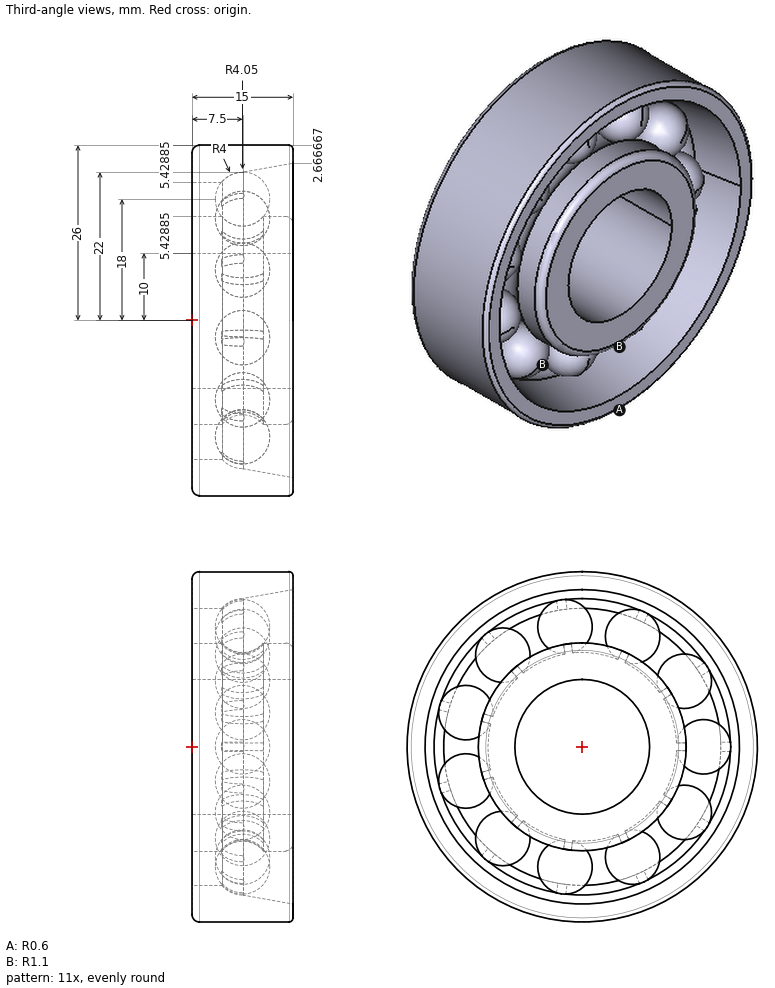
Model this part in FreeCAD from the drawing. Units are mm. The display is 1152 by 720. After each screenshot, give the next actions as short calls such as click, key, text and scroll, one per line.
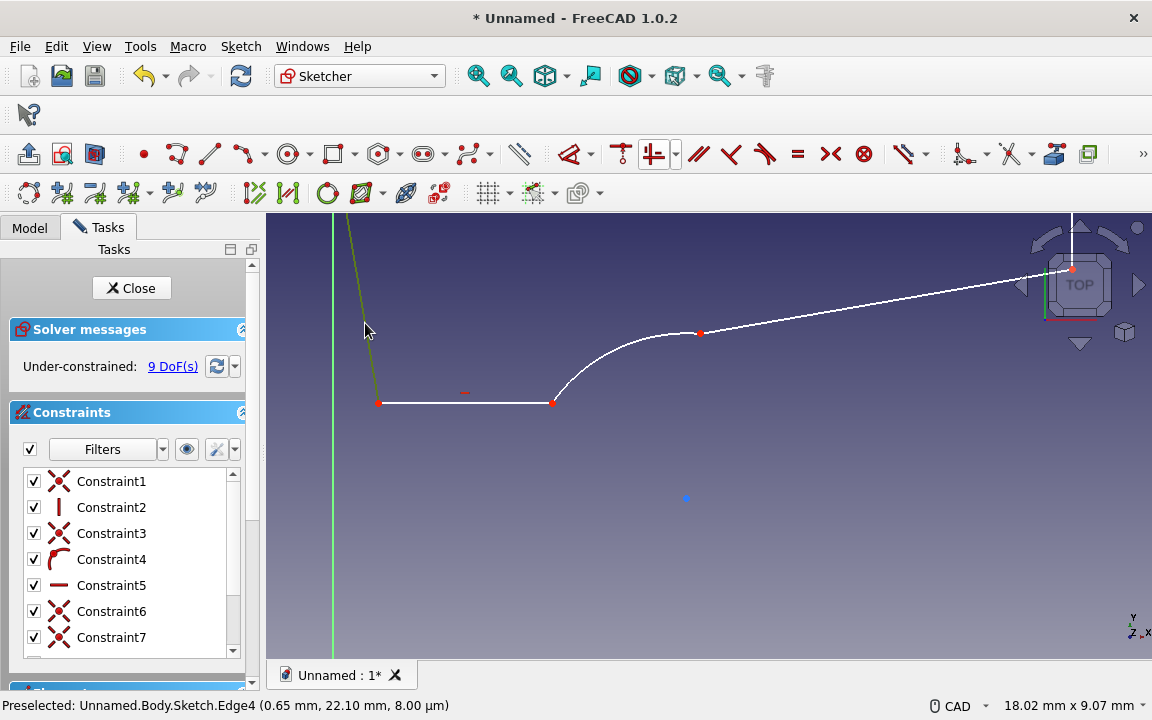
key(v)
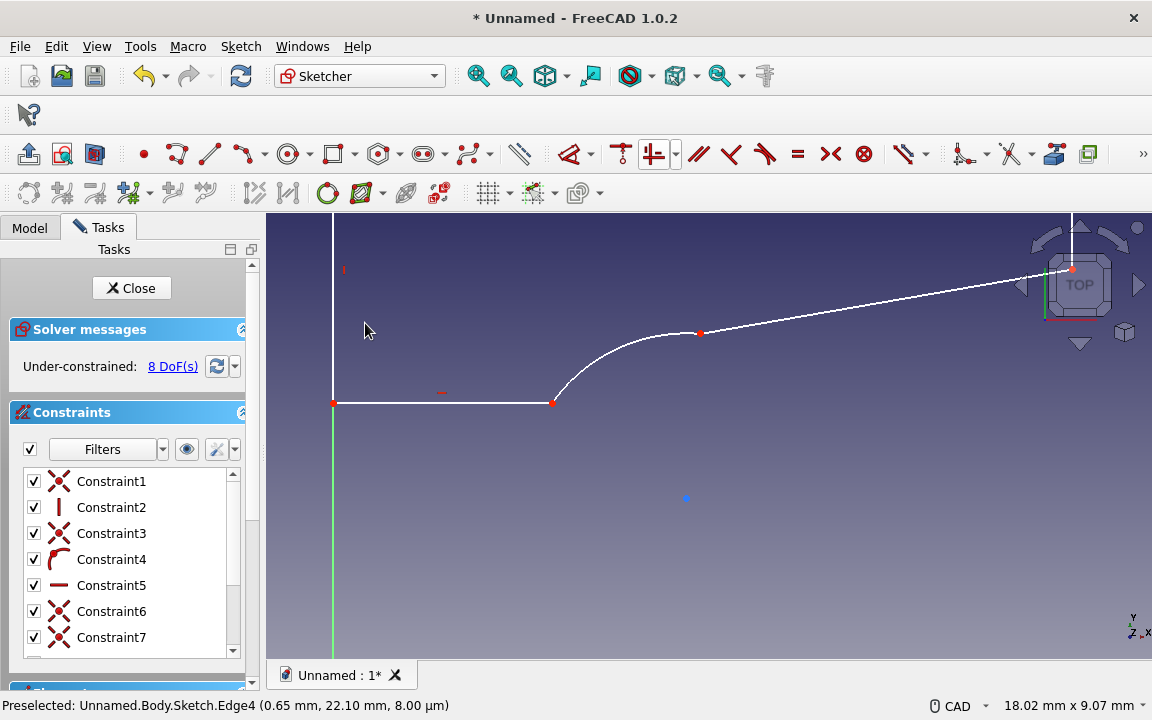
click(568, 154)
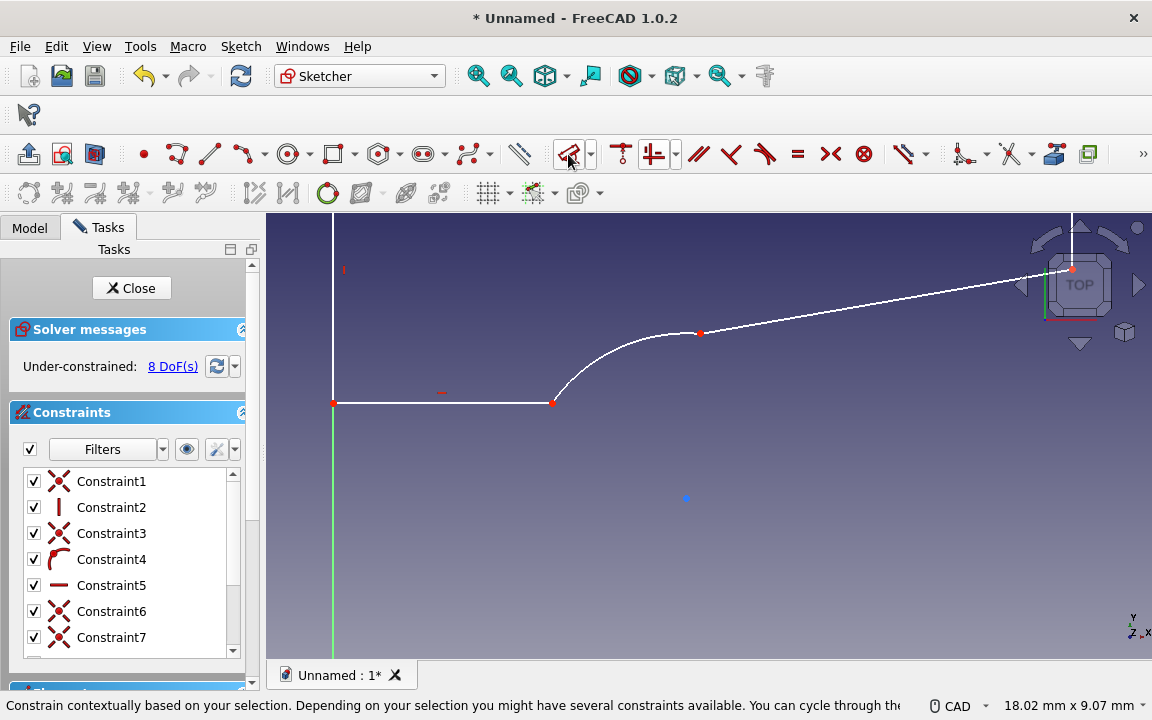
scroll(625, 351, down, 8)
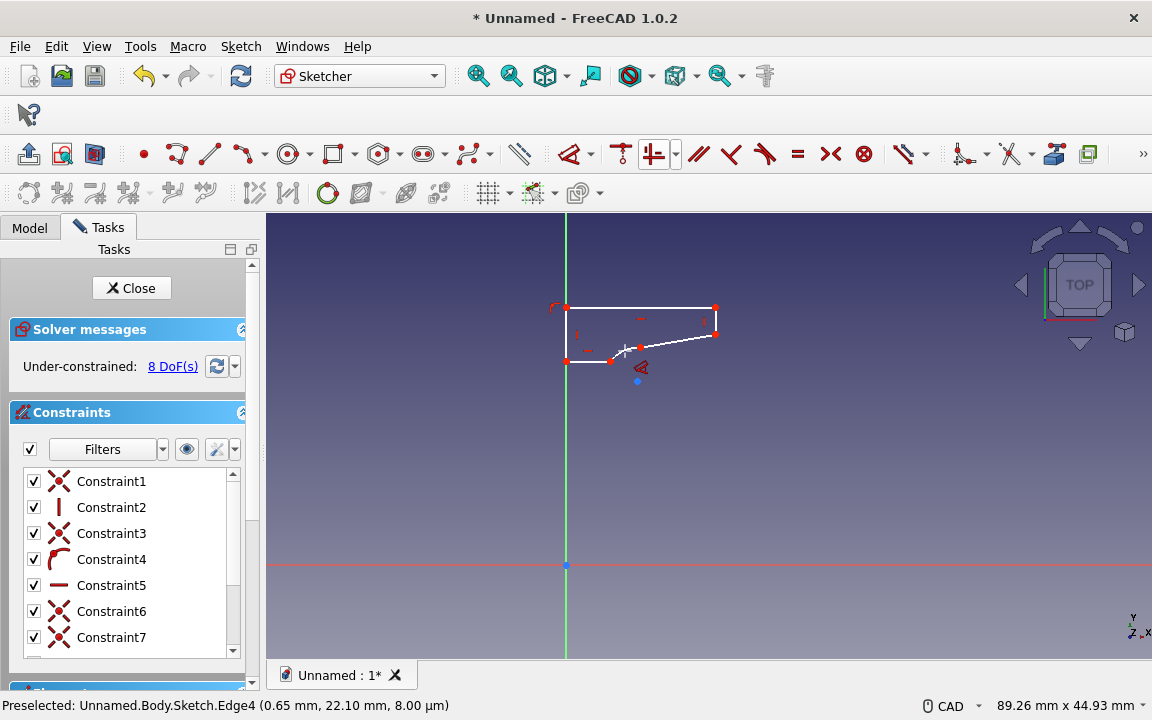
scroll(630, 349, up, 2)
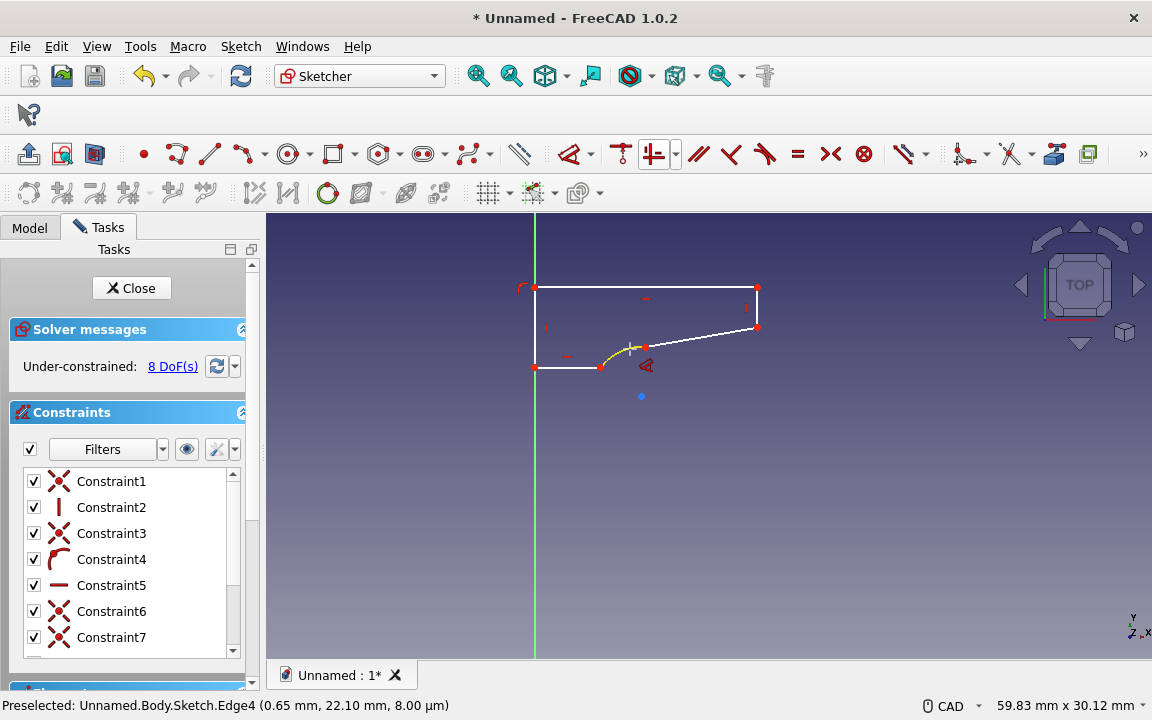
click(630, 348)
click(623, 317)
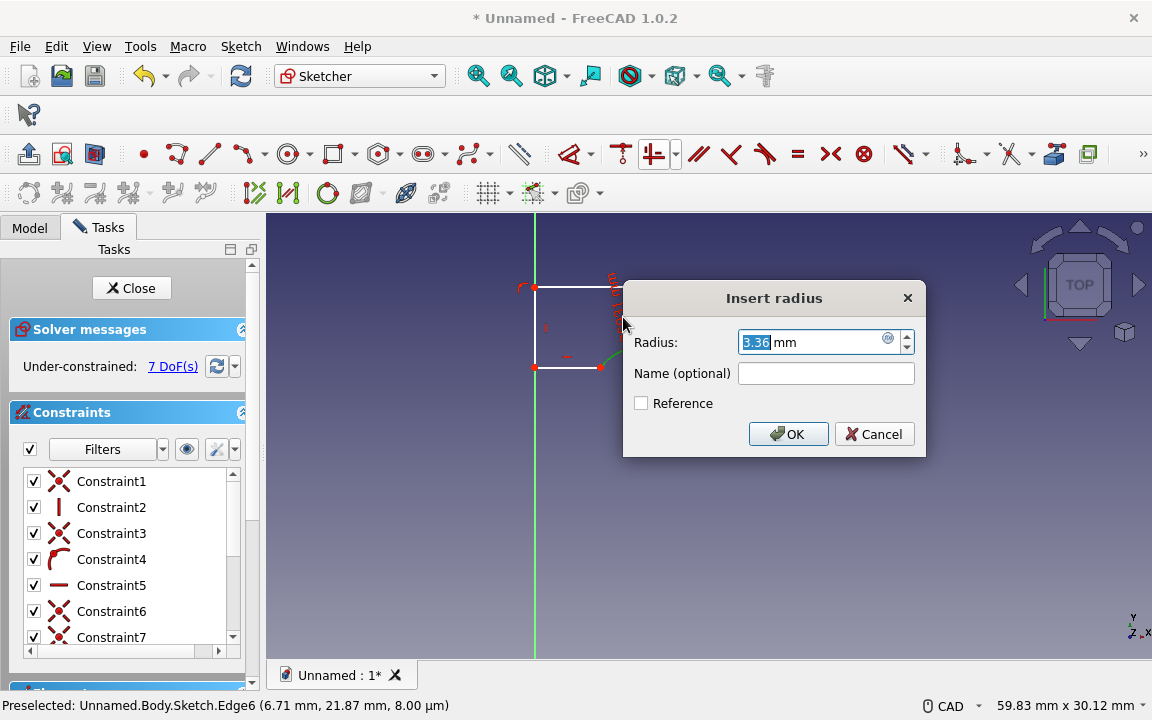
text(4)
key(Return)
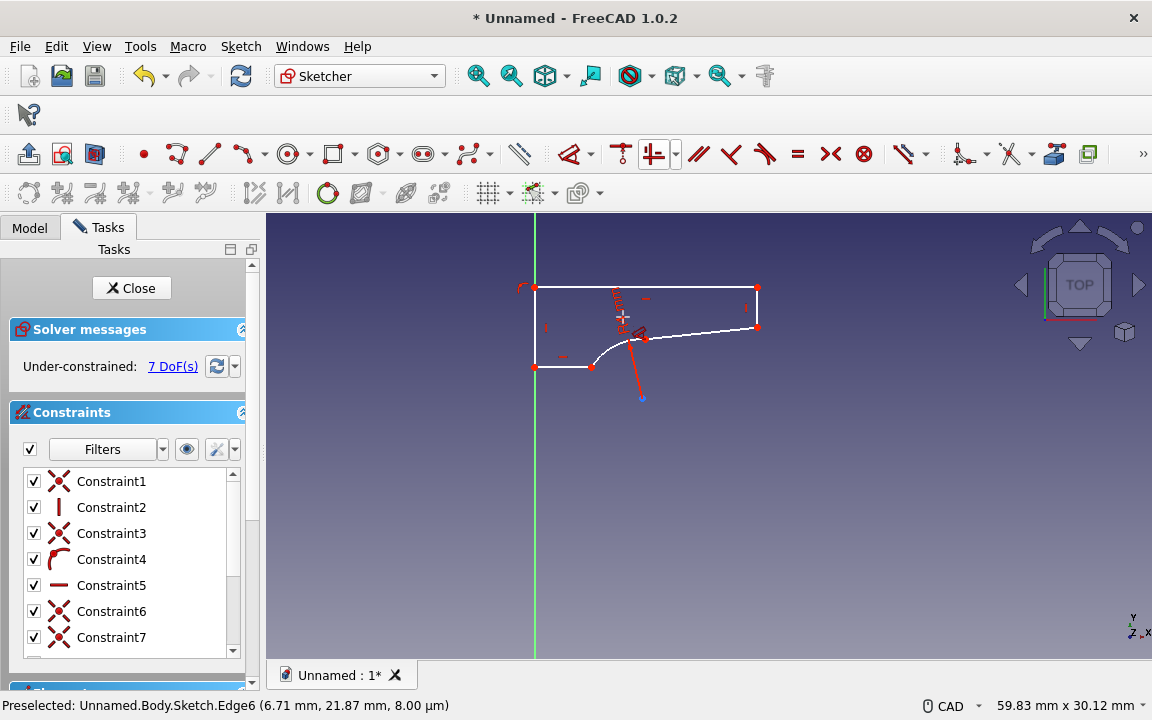
click(691, 287)
click(646, 253)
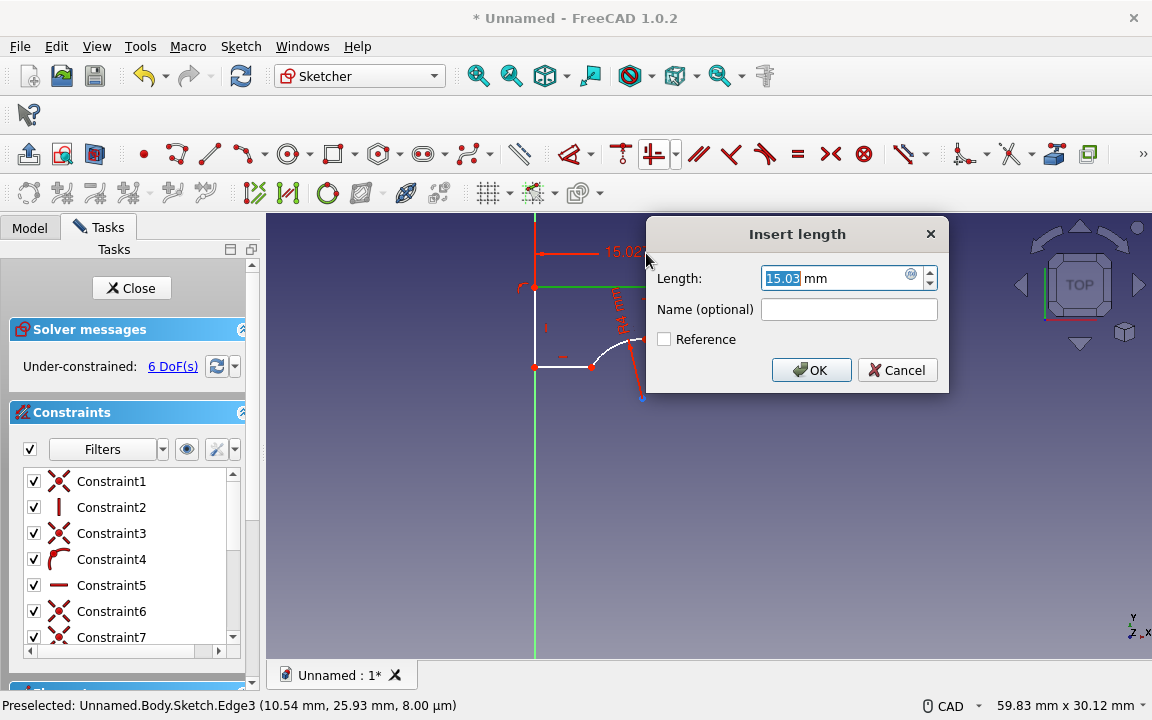
text(15)
key(Return)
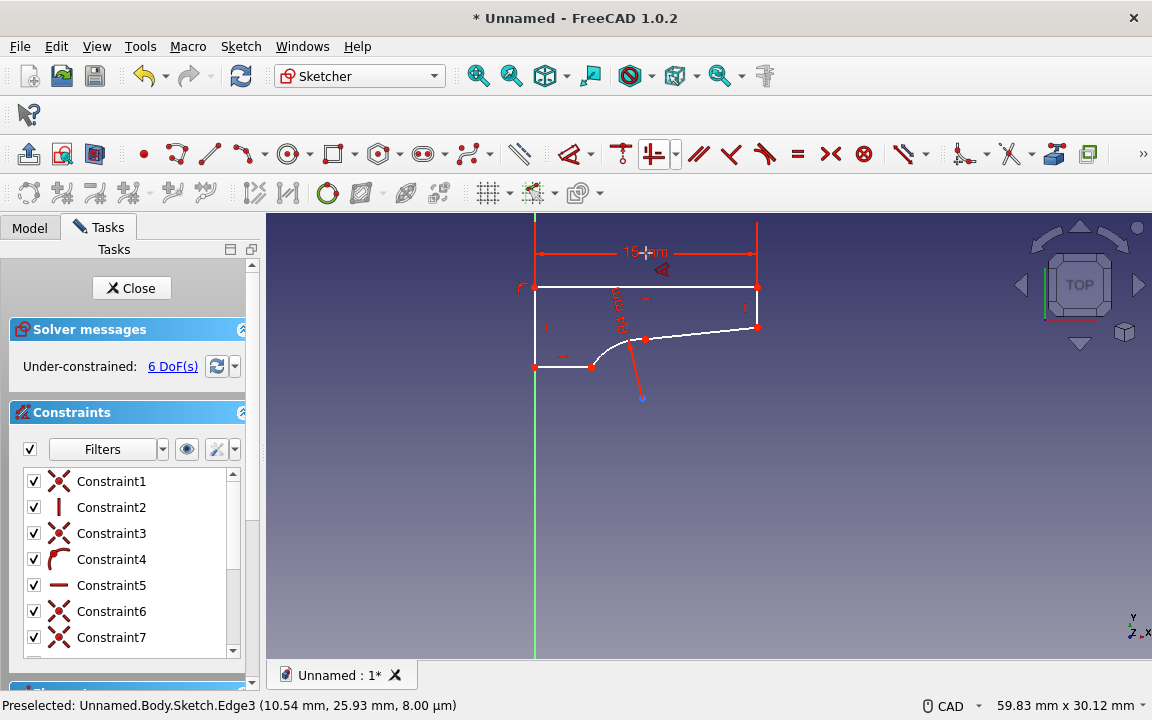
click(646, 339)
click(501, 485)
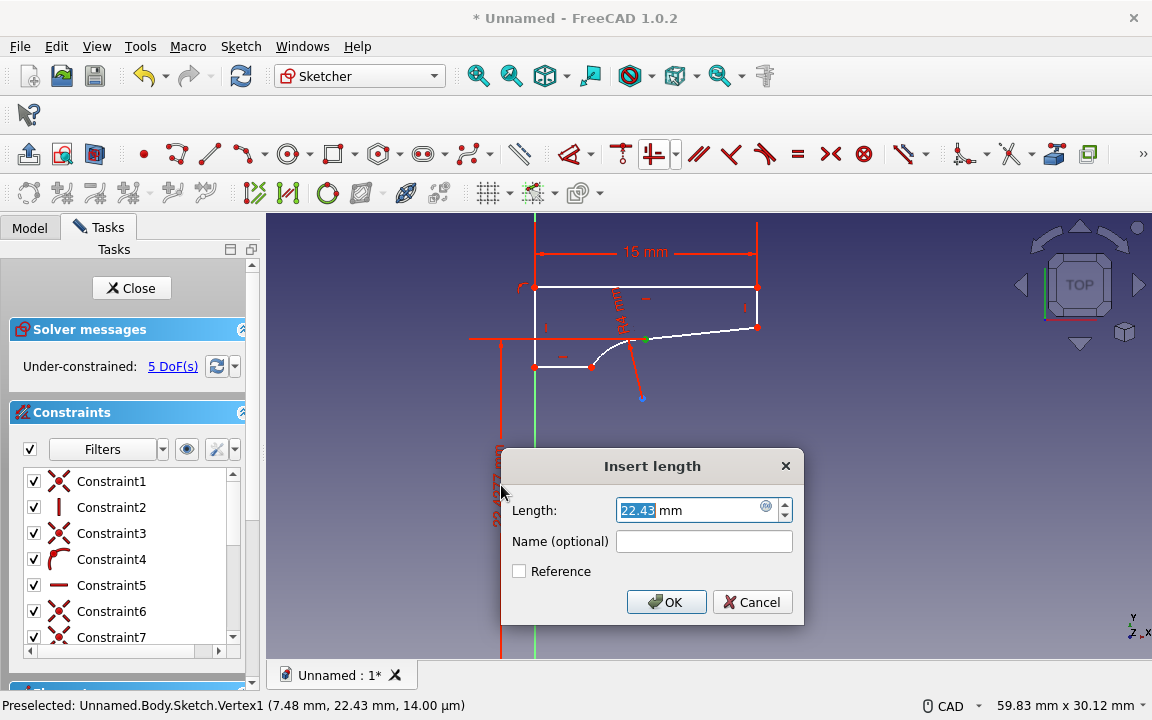
text(22)
key(Return)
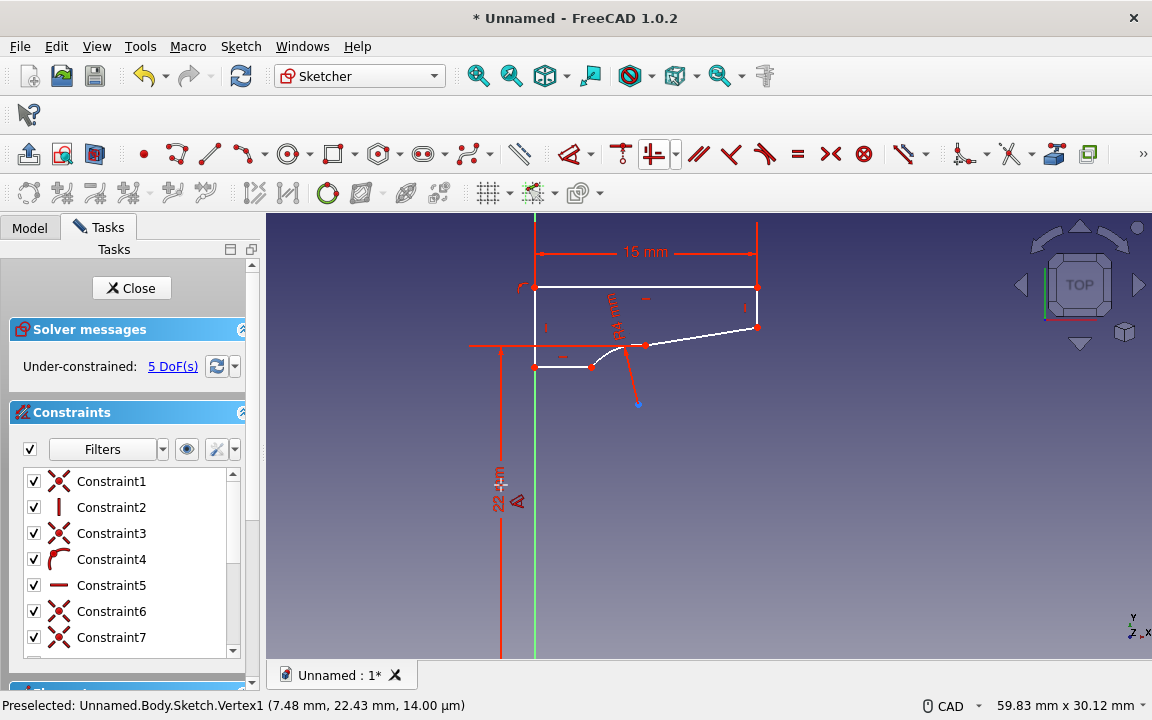
click(757, 287)
click(791, 459)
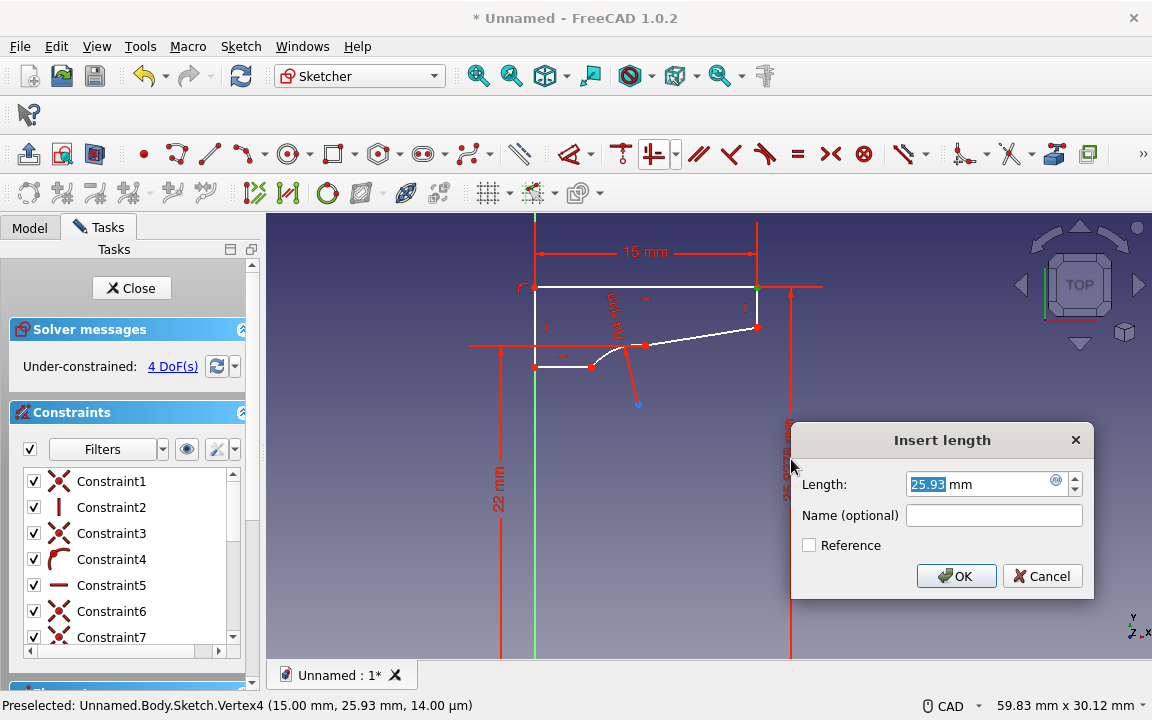
text(26)
key(Return)